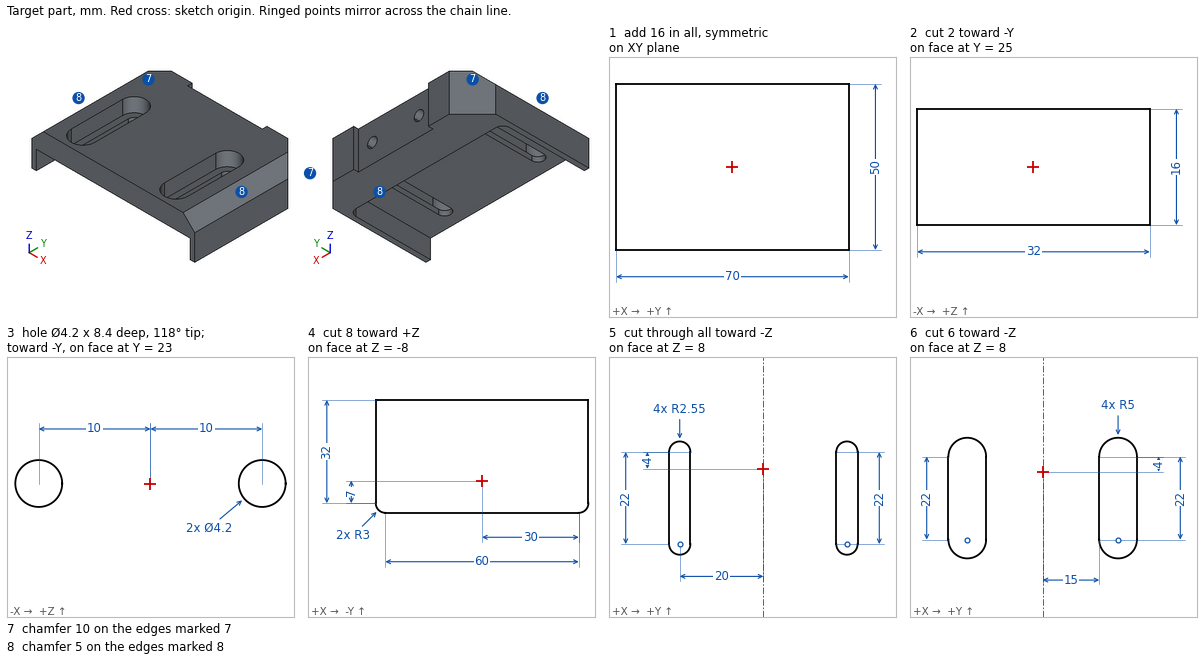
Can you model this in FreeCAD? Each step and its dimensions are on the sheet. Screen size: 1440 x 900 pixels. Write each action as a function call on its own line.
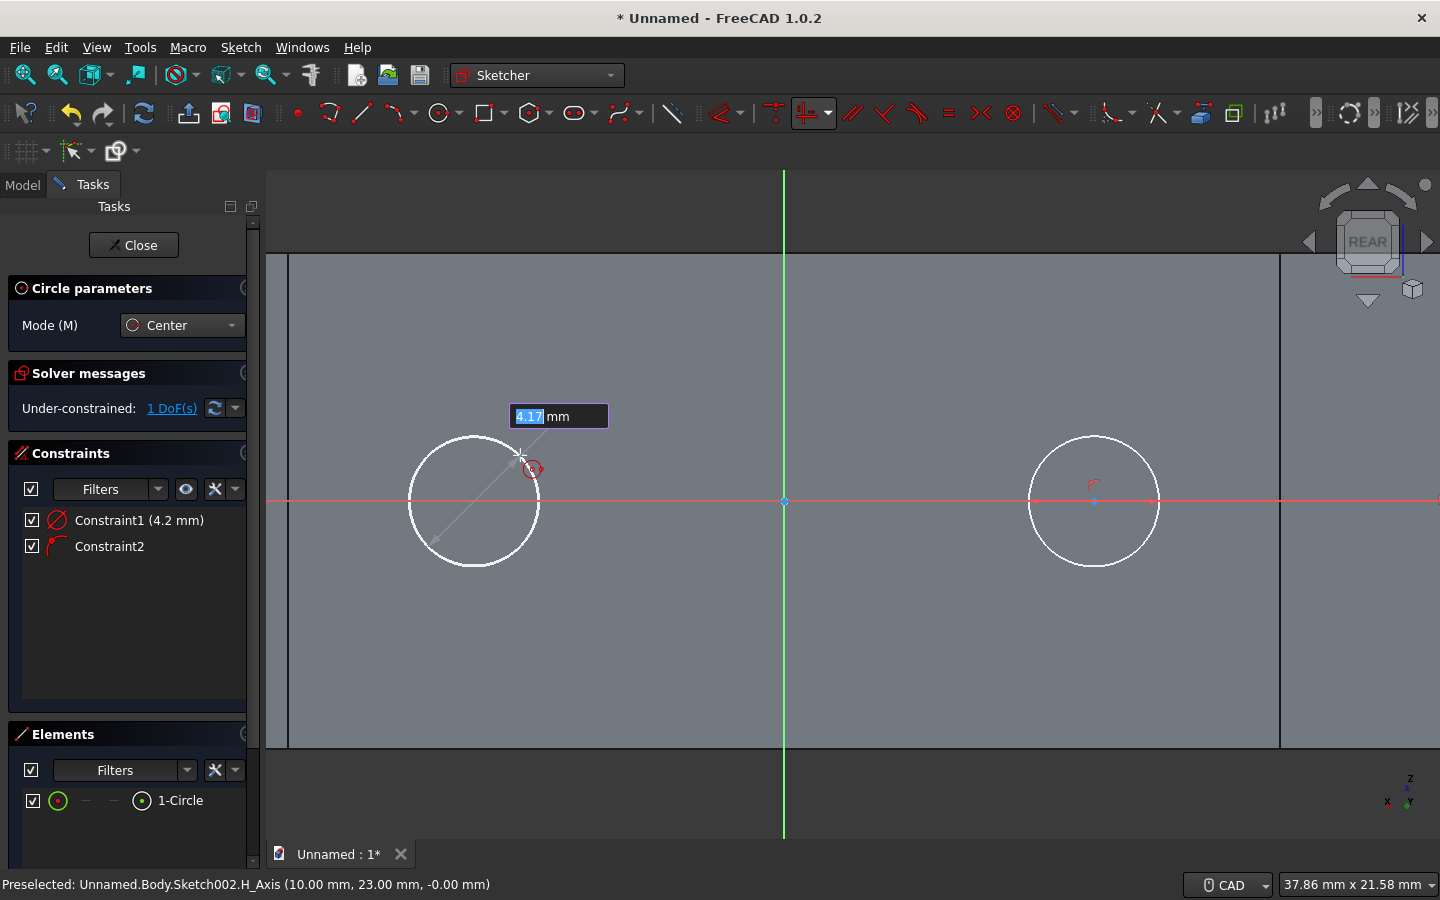
text(4.2)
key(Return)
key(Escape)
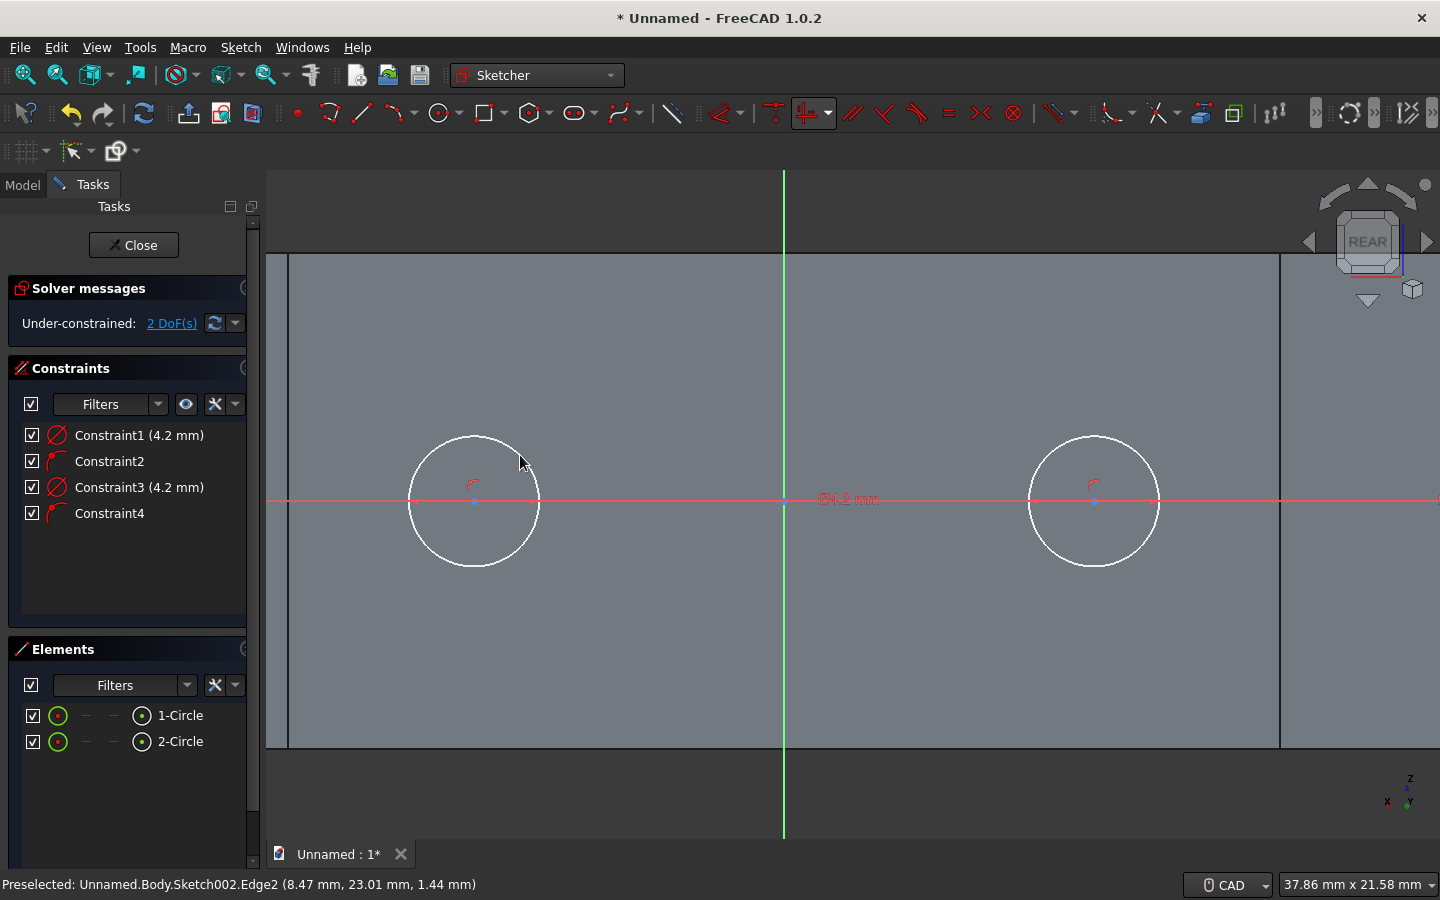
click(720, 114)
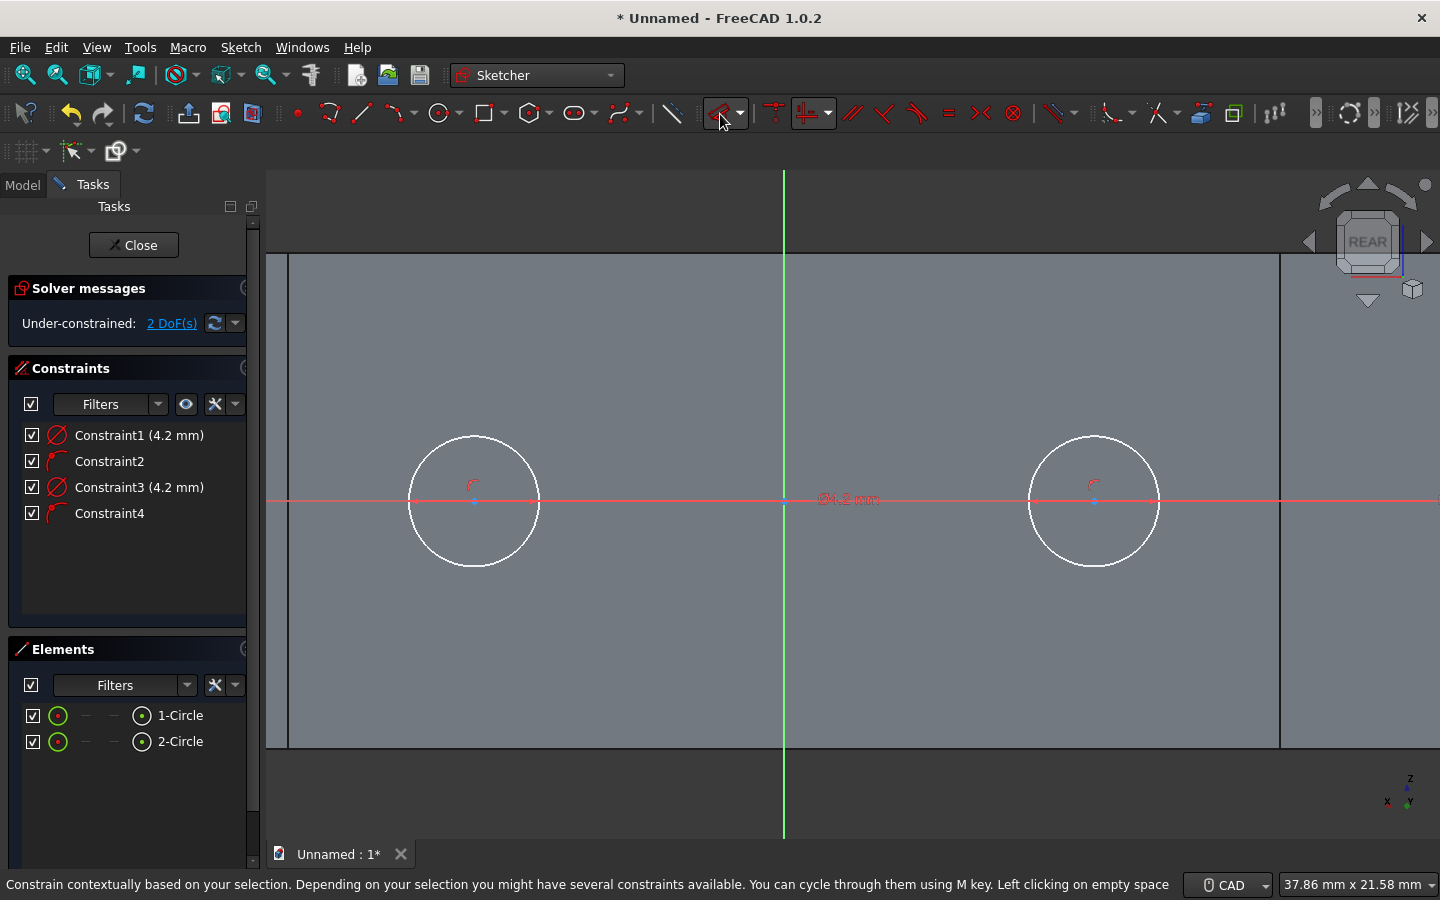
click(1094, 501)
click(939, 535)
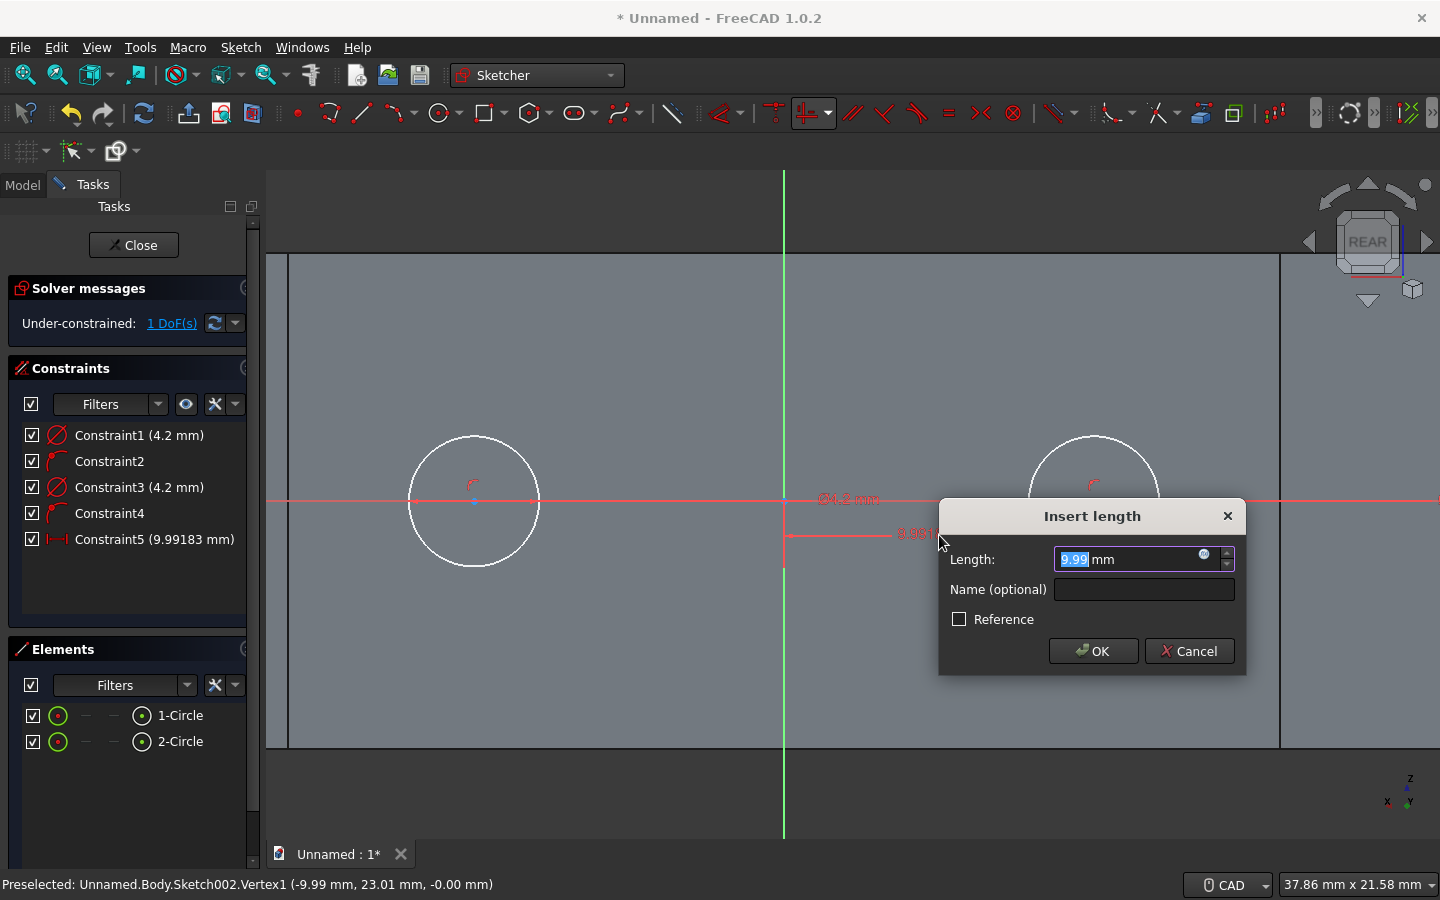
text(10)
key(Return)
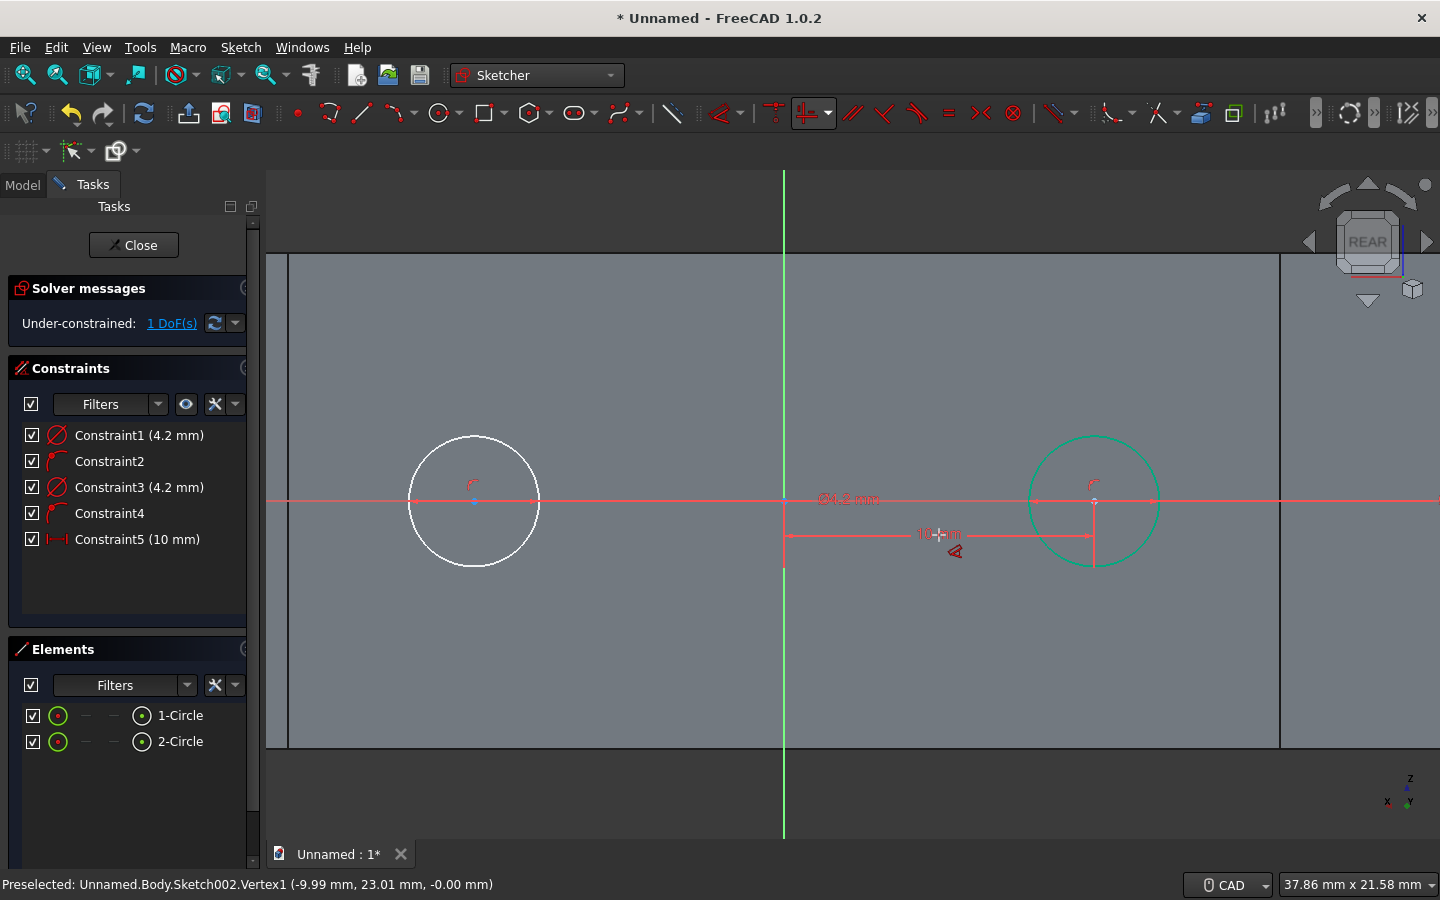
click(474, 501)
click(629, 535)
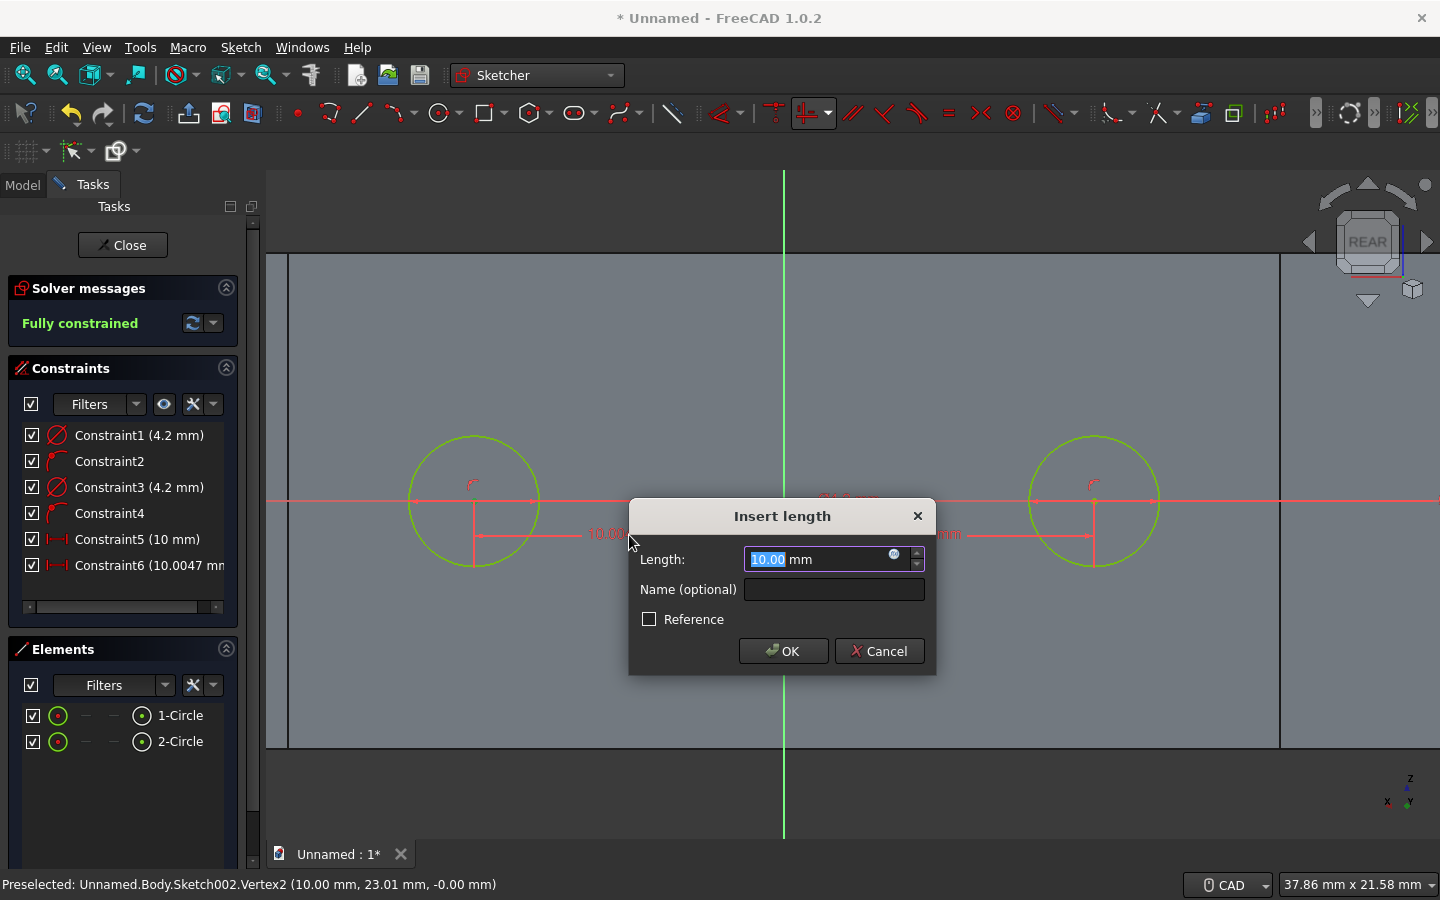
text(10)
key(Return)
key(Escape)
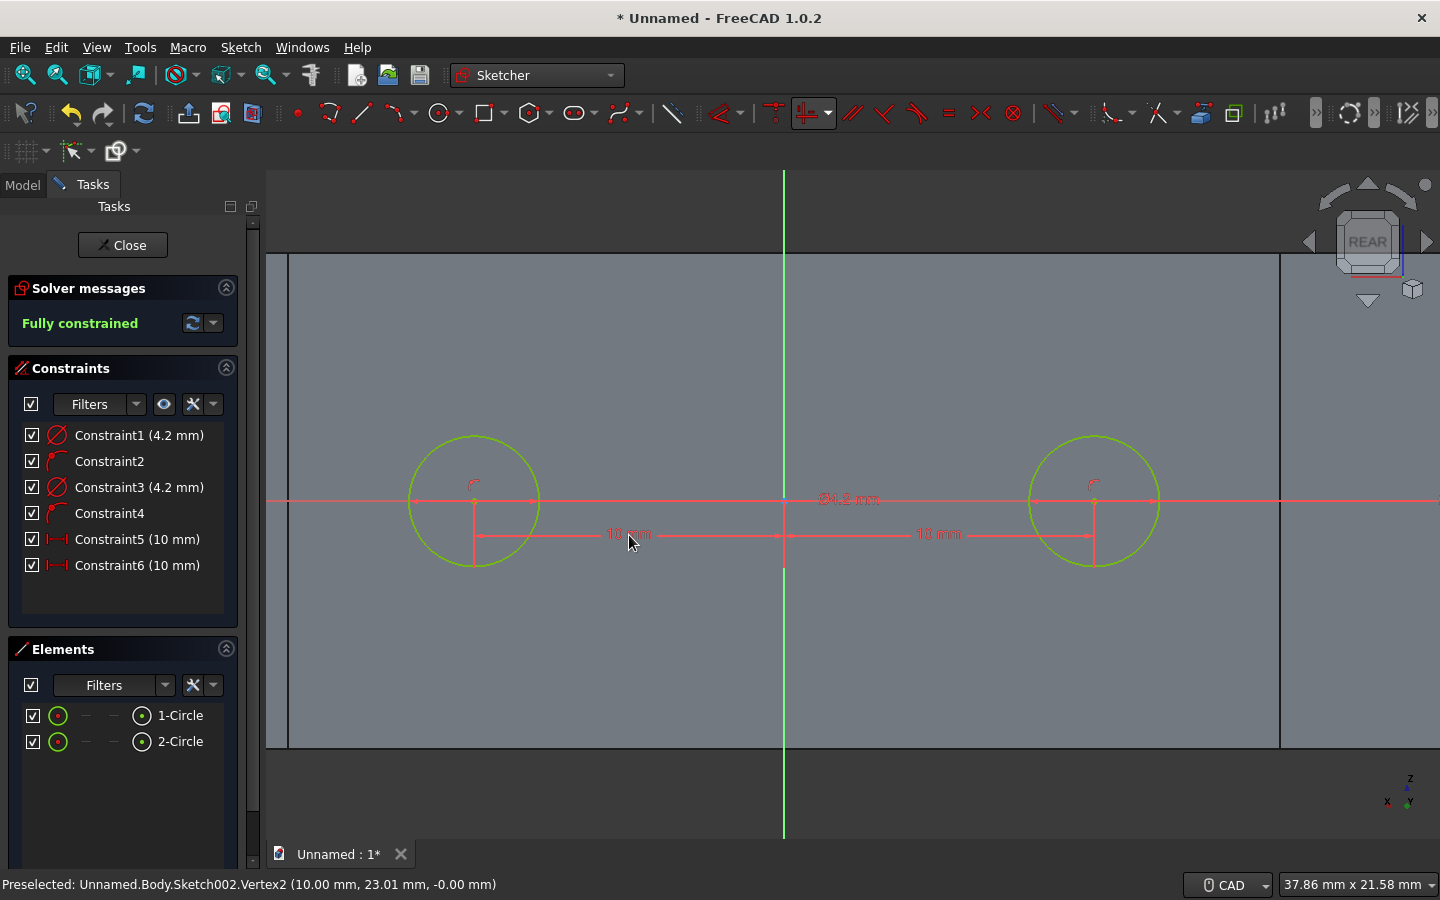
click(123, 245)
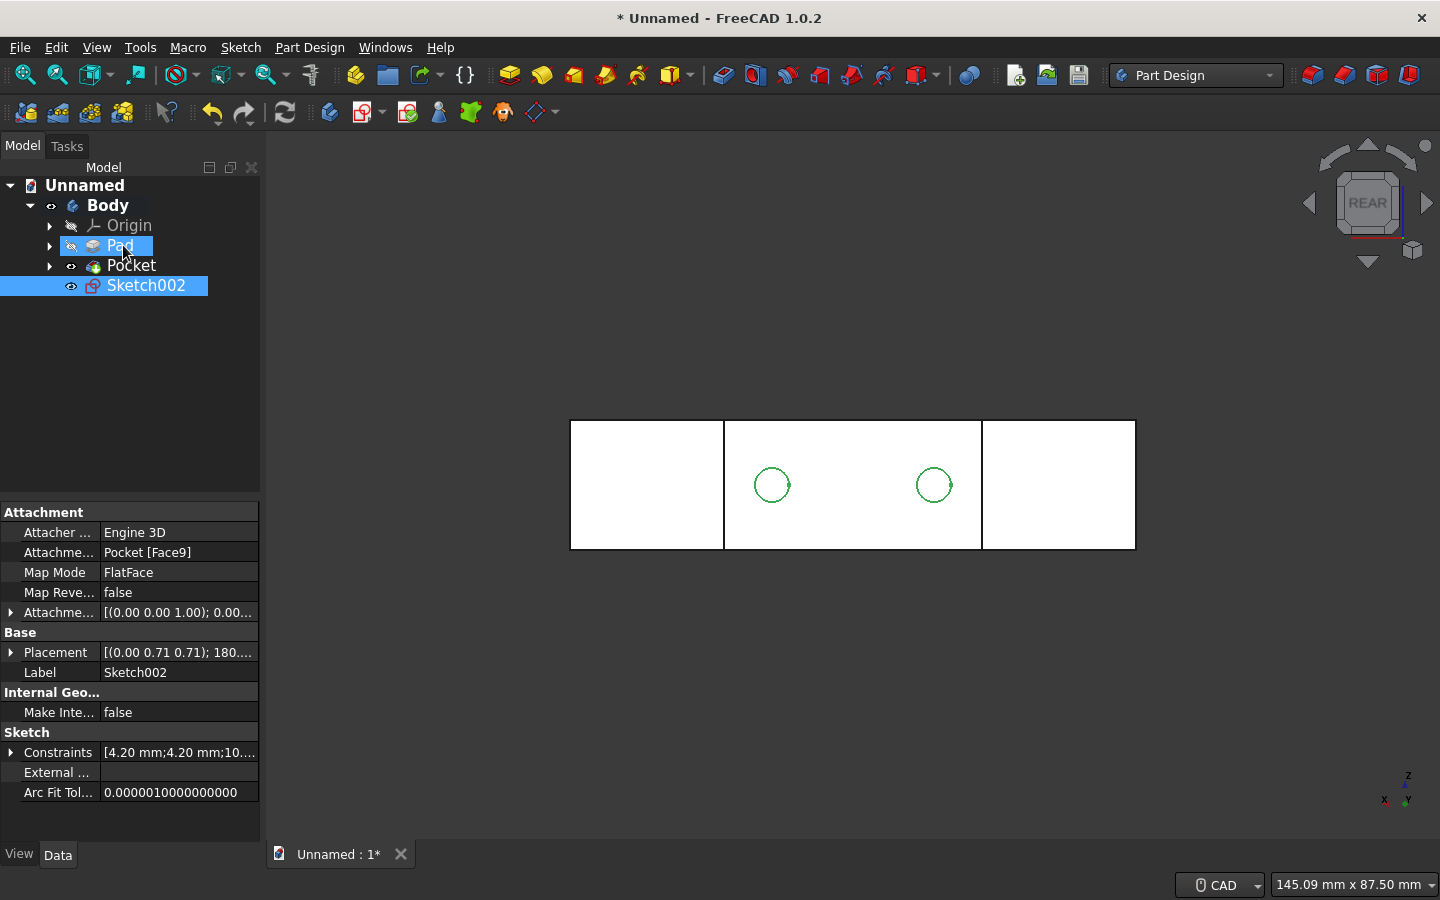
click(756, 76)